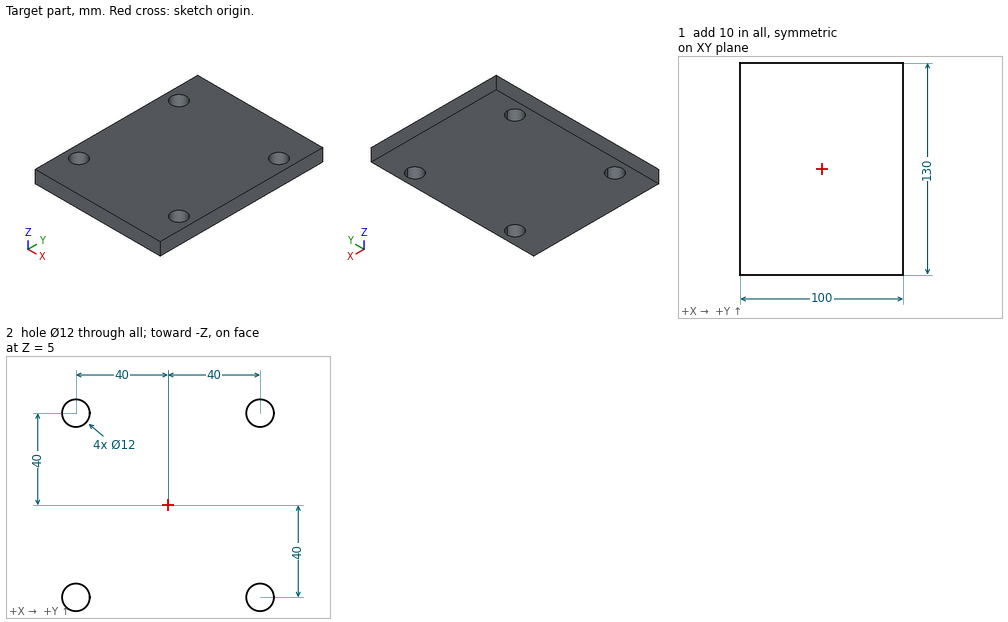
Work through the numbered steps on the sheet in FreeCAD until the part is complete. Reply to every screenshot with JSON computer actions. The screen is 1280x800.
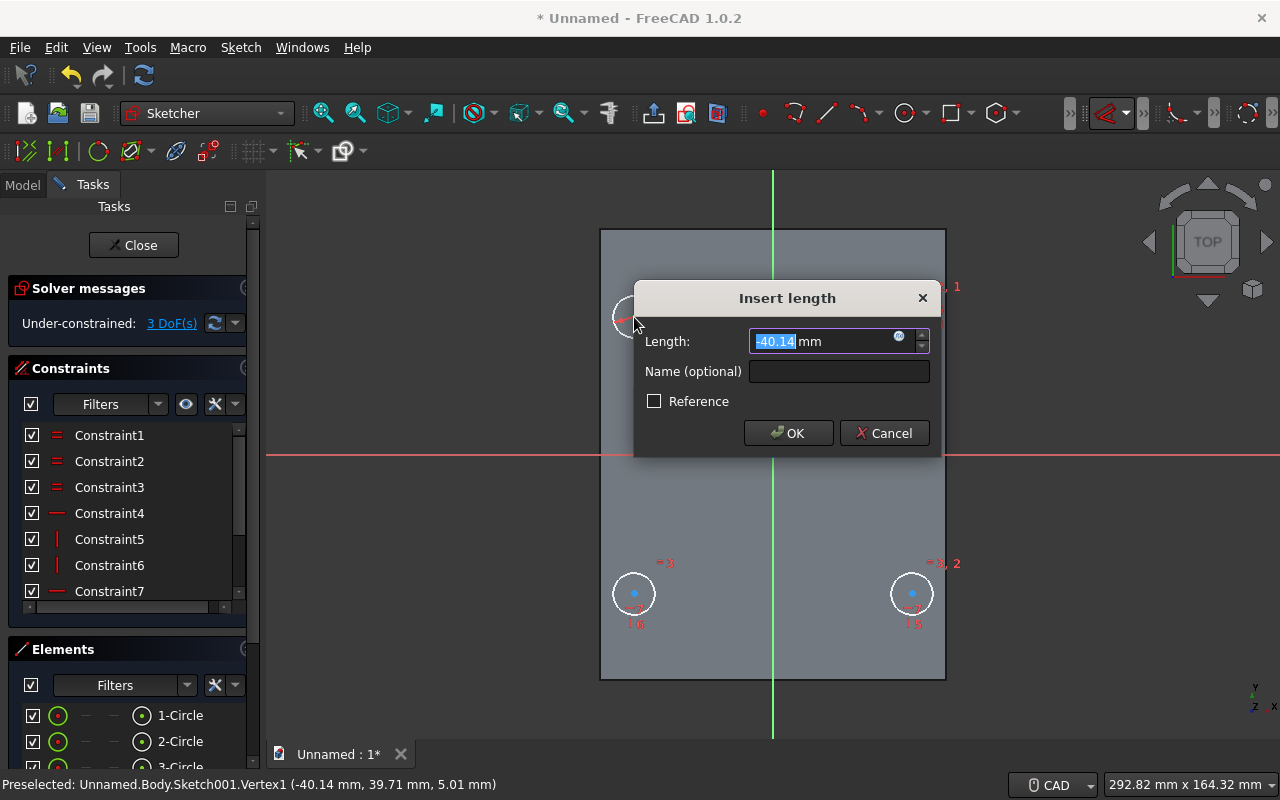
{"action": "type", "text": "-40"}
{"action": "key", "text": "Return"}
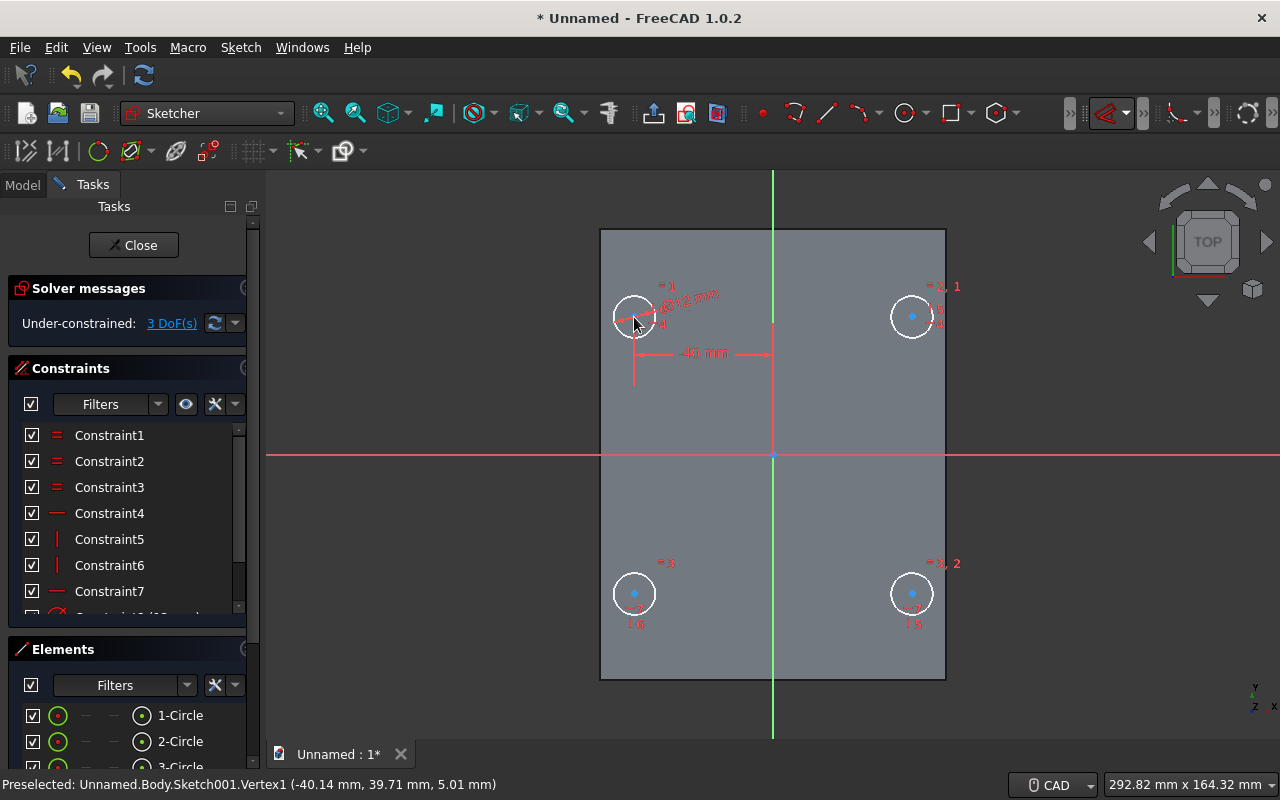
{"action": "left_click", "coordinate": [634, 317]}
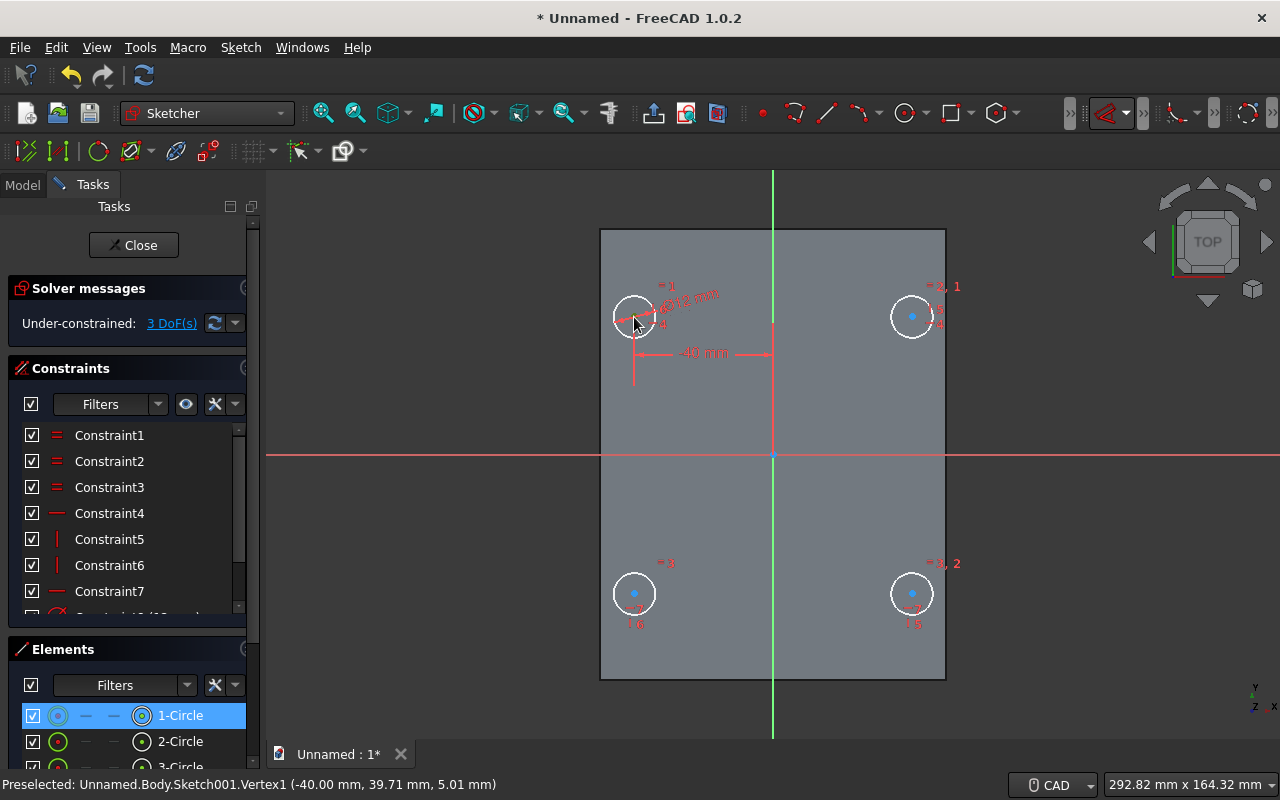
{"action": "key", "text": "i"}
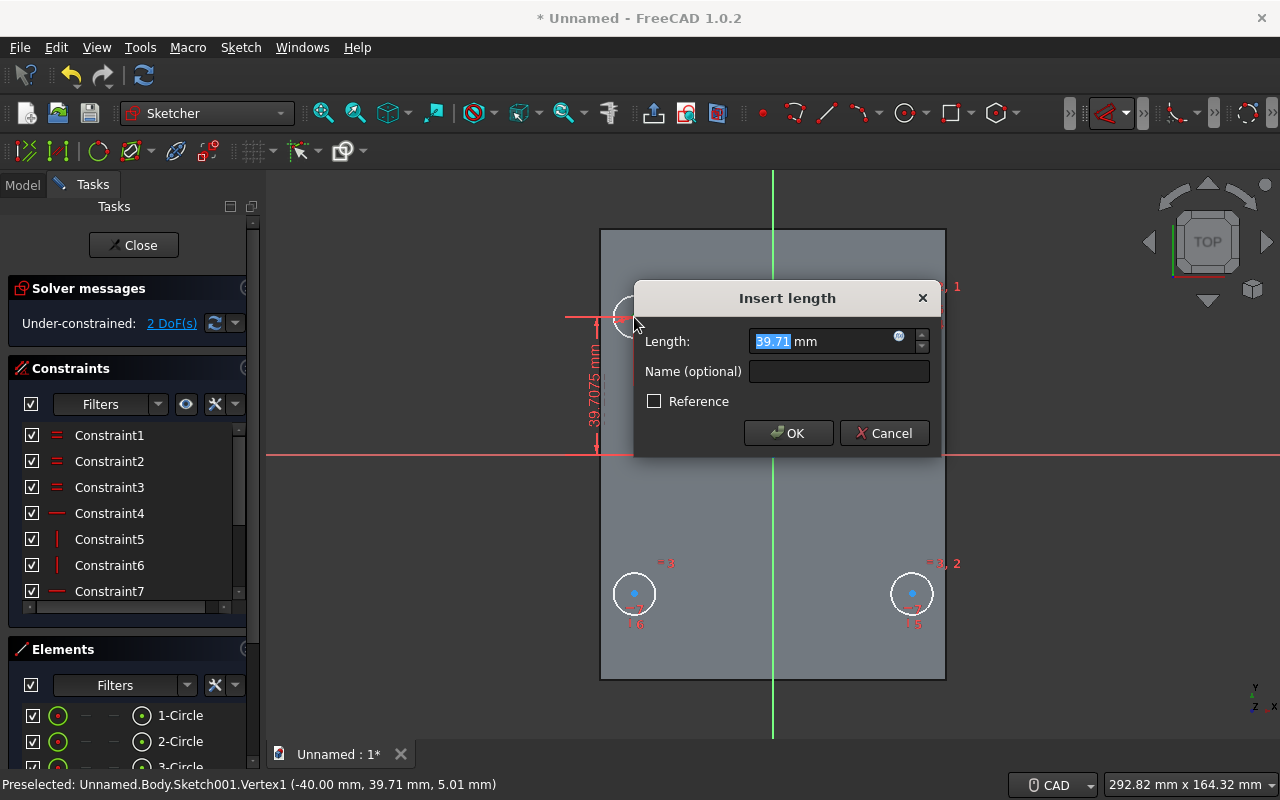
{"action": "type", "text": "40"}
{"action": "key", "text": "Return"}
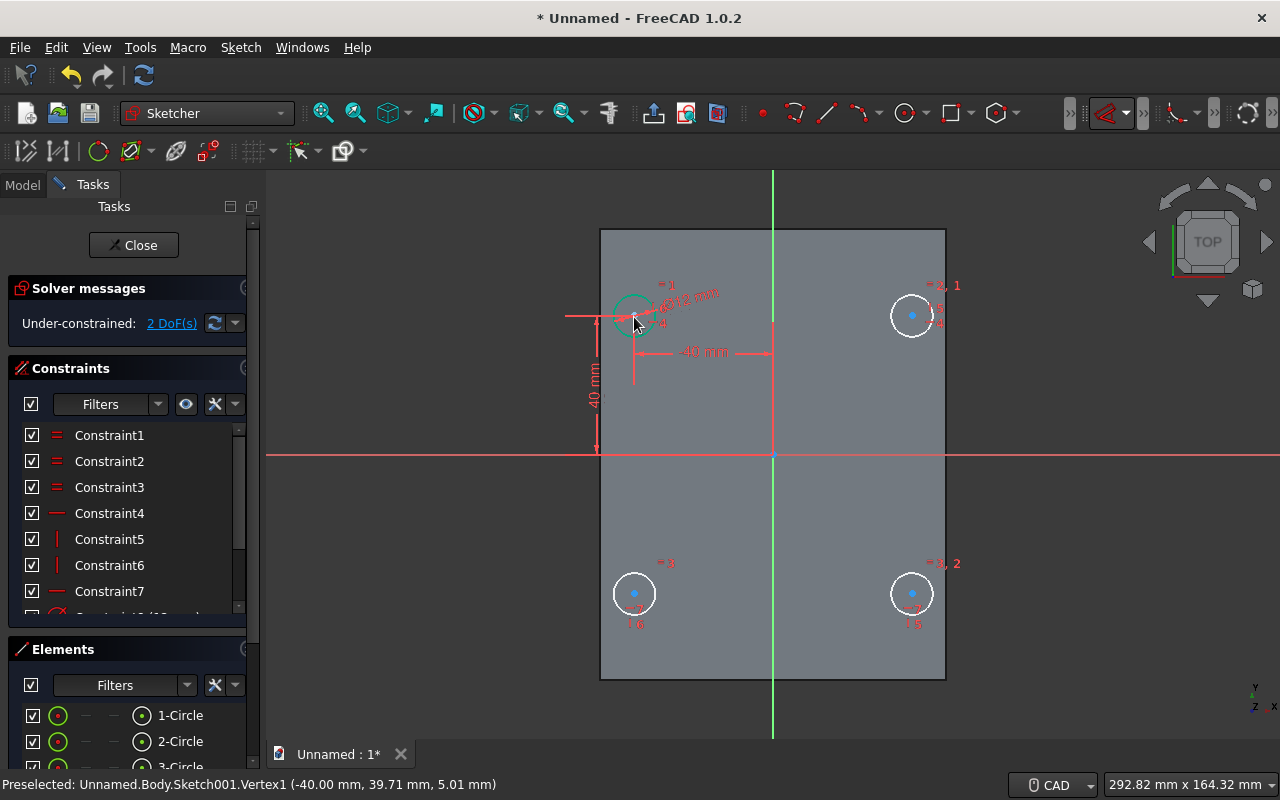
{"action": "left_click", "coordinate": [912, 316]}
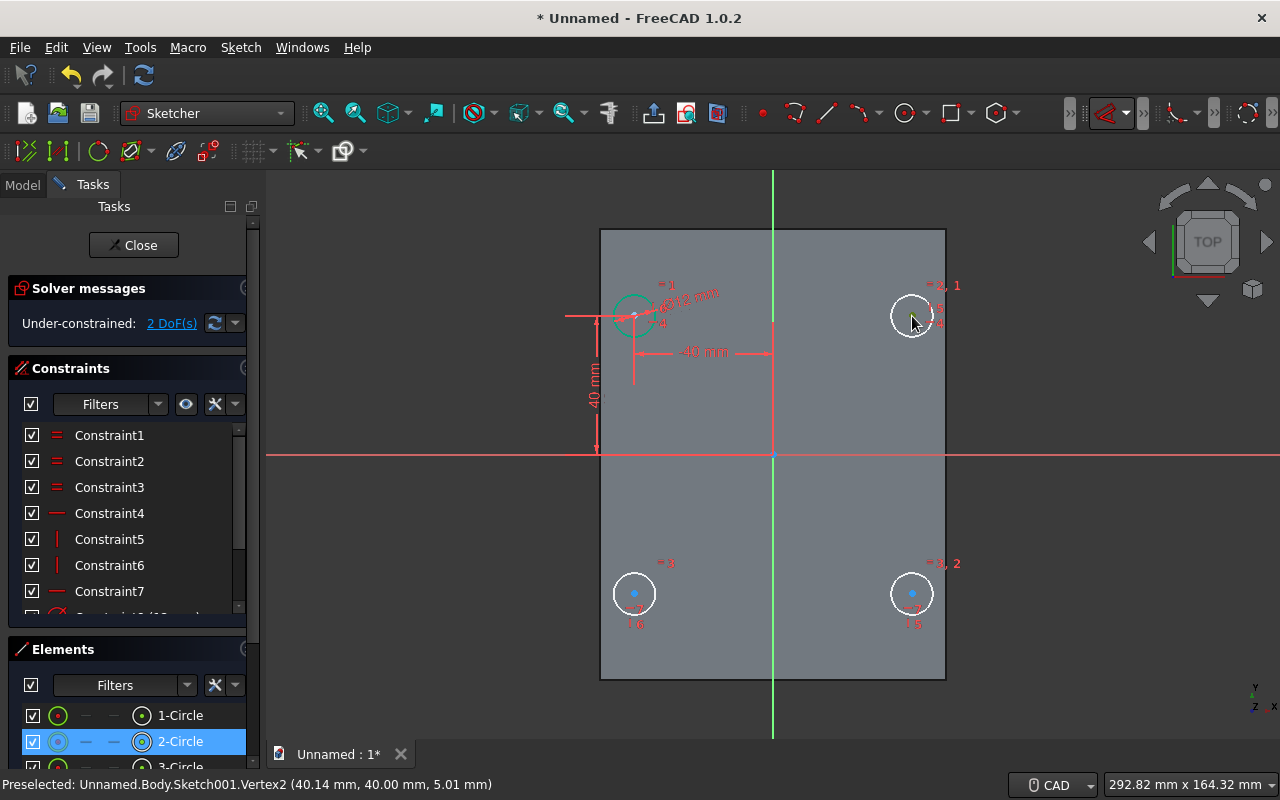
{"action": "key", "text": "l"}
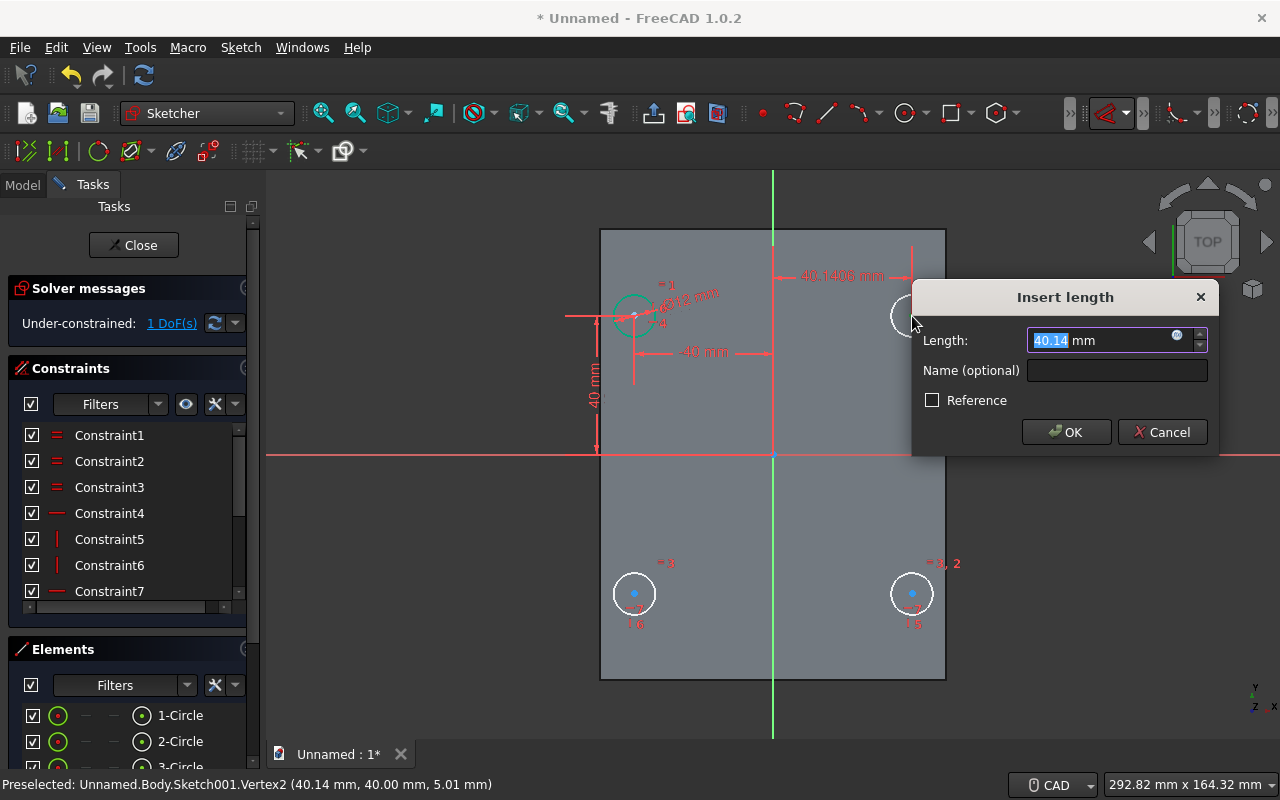
{"action": "type", "text": "40"}
{"action": "key", "text": "Return"}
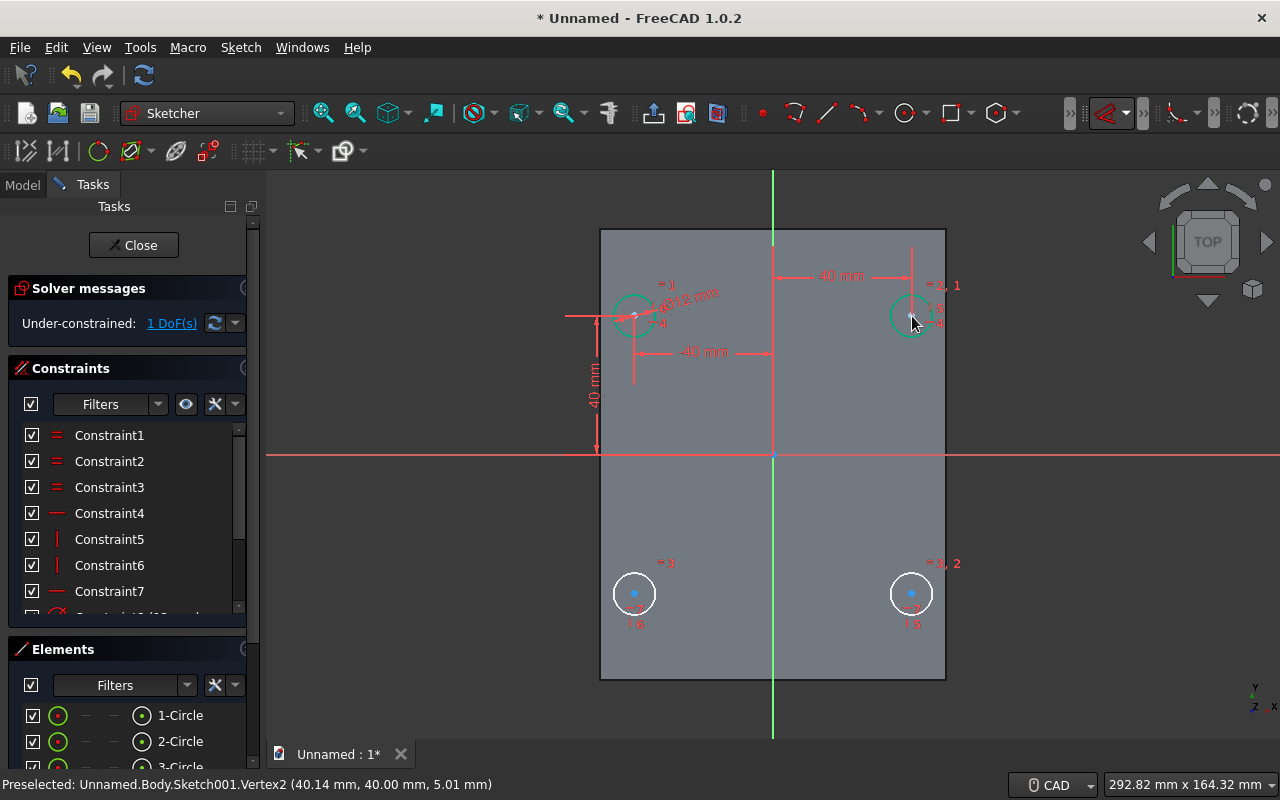
{"action": "left_click", "coordinate": [912, 594]}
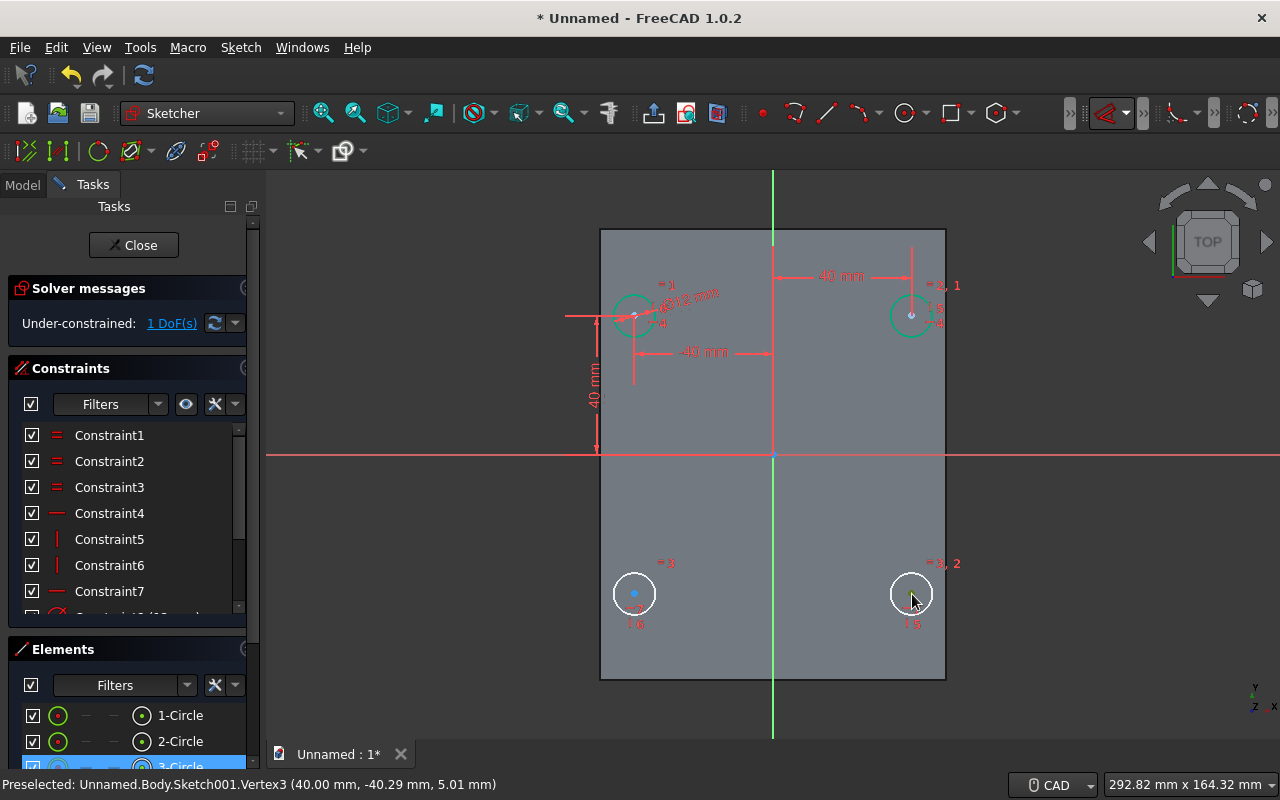
{"action": "left_click", "coordinate": [1128, 114]}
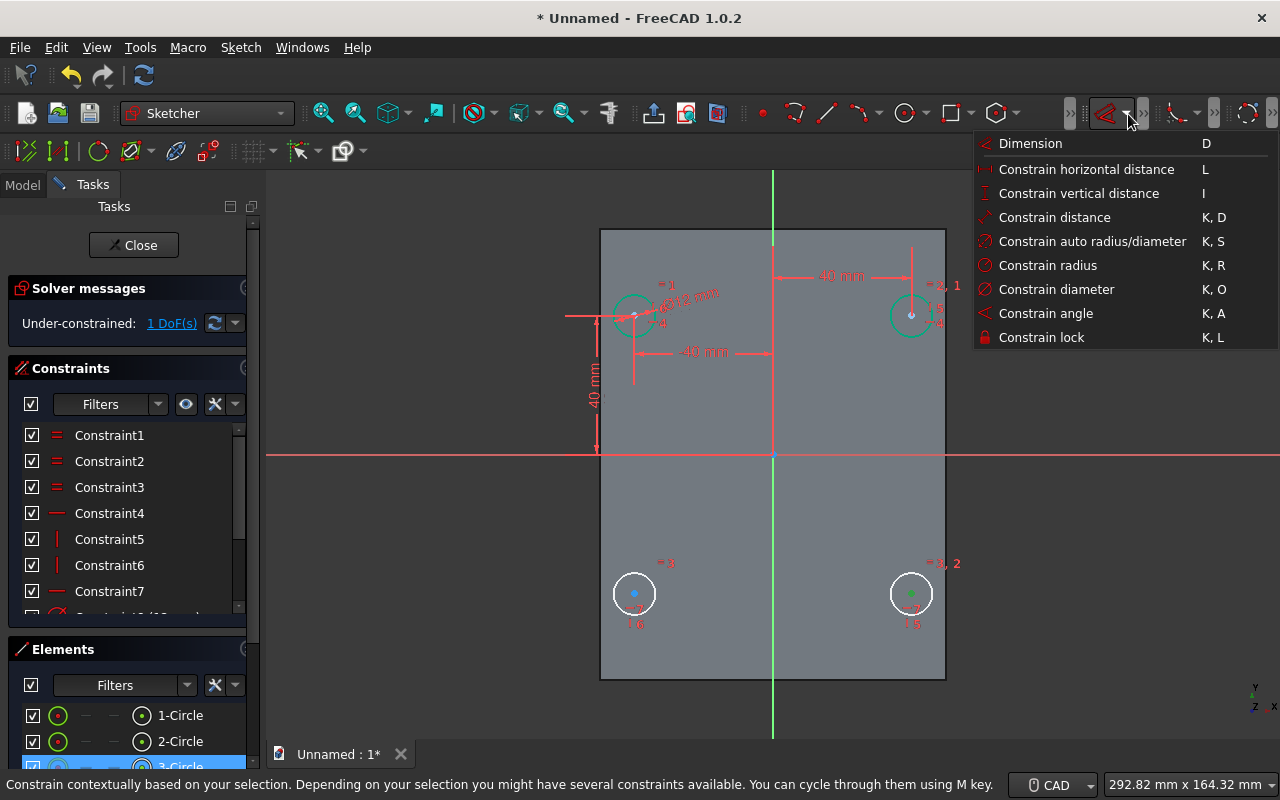
{"action": "left_click", "coordinate": [1126, 193]}